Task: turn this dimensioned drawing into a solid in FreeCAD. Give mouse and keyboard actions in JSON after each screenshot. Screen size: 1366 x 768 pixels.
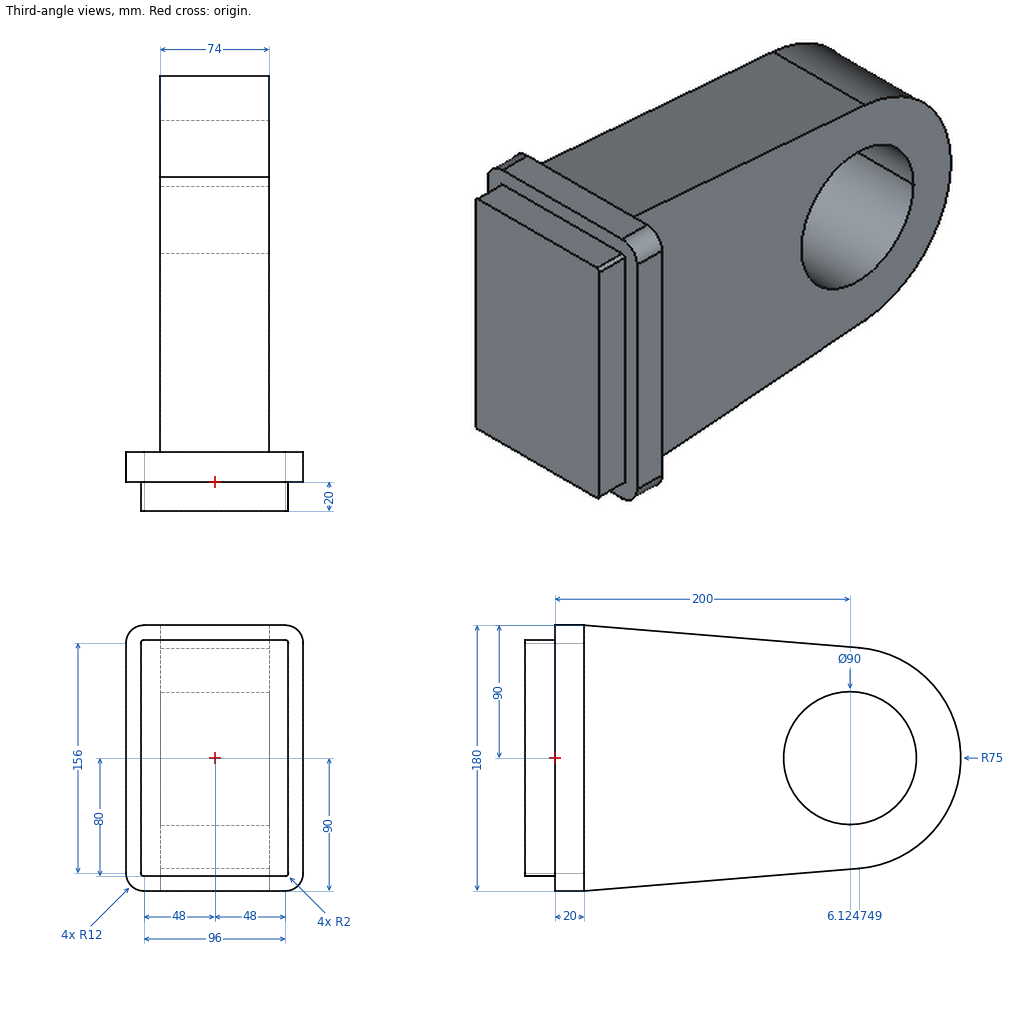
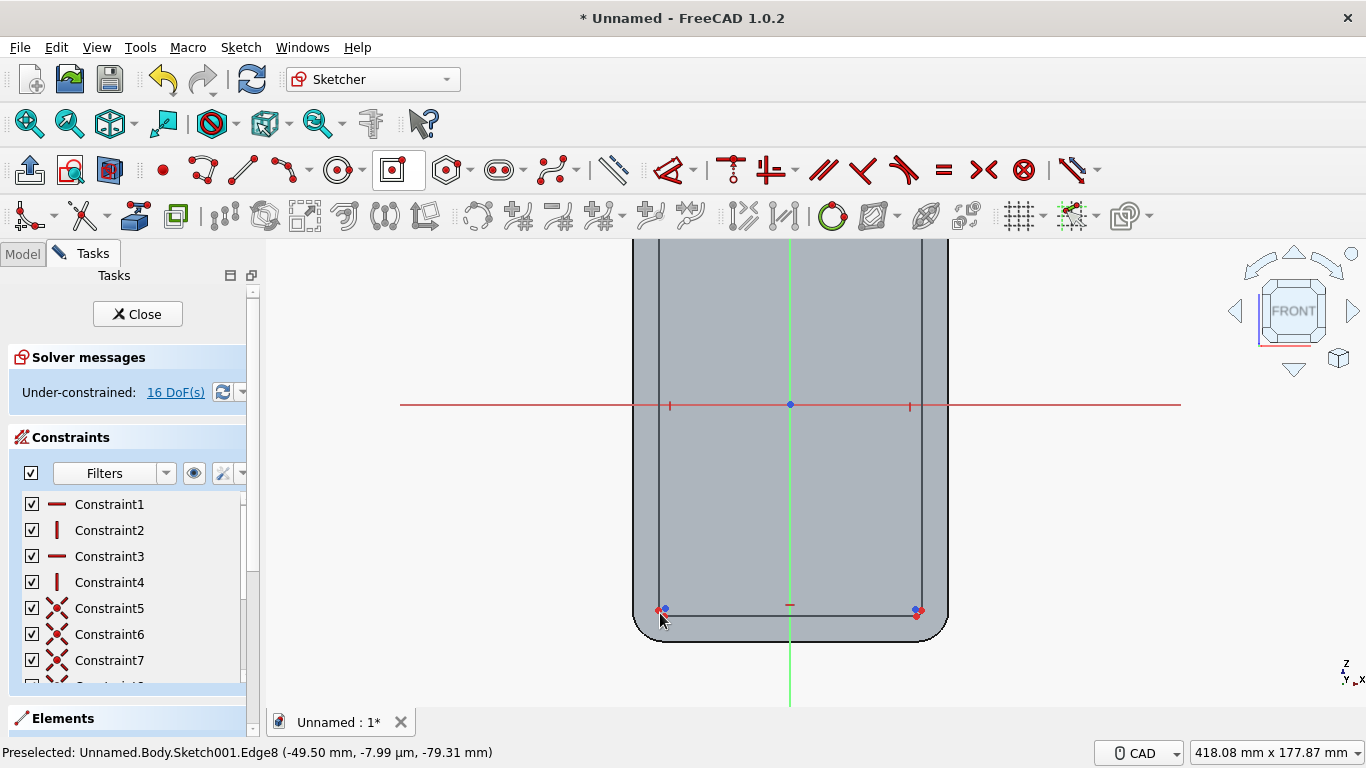
{"action": "left_click", "coordinate": [714, 615]}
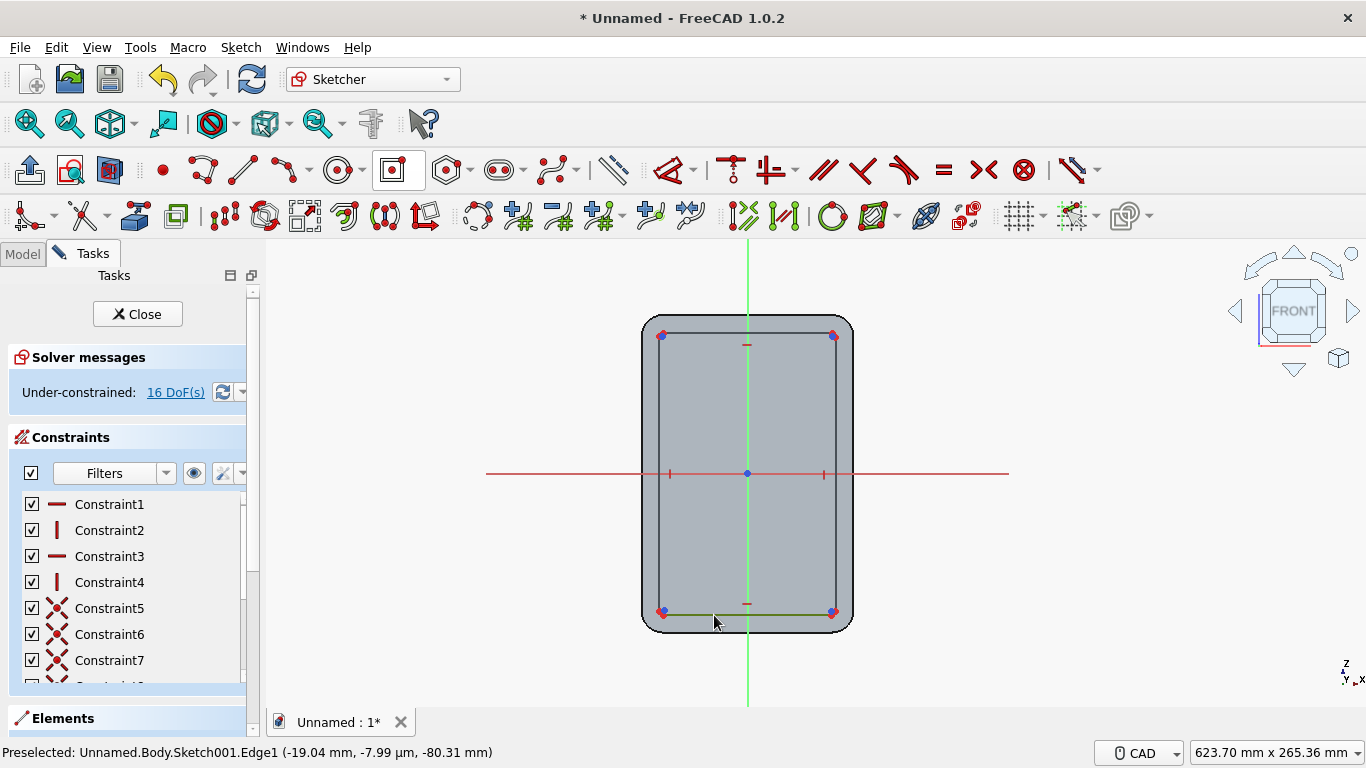
{"action": "scroll", "coordinate": [834, 614], "scroll_direction": "up", "scroll_amount": 9}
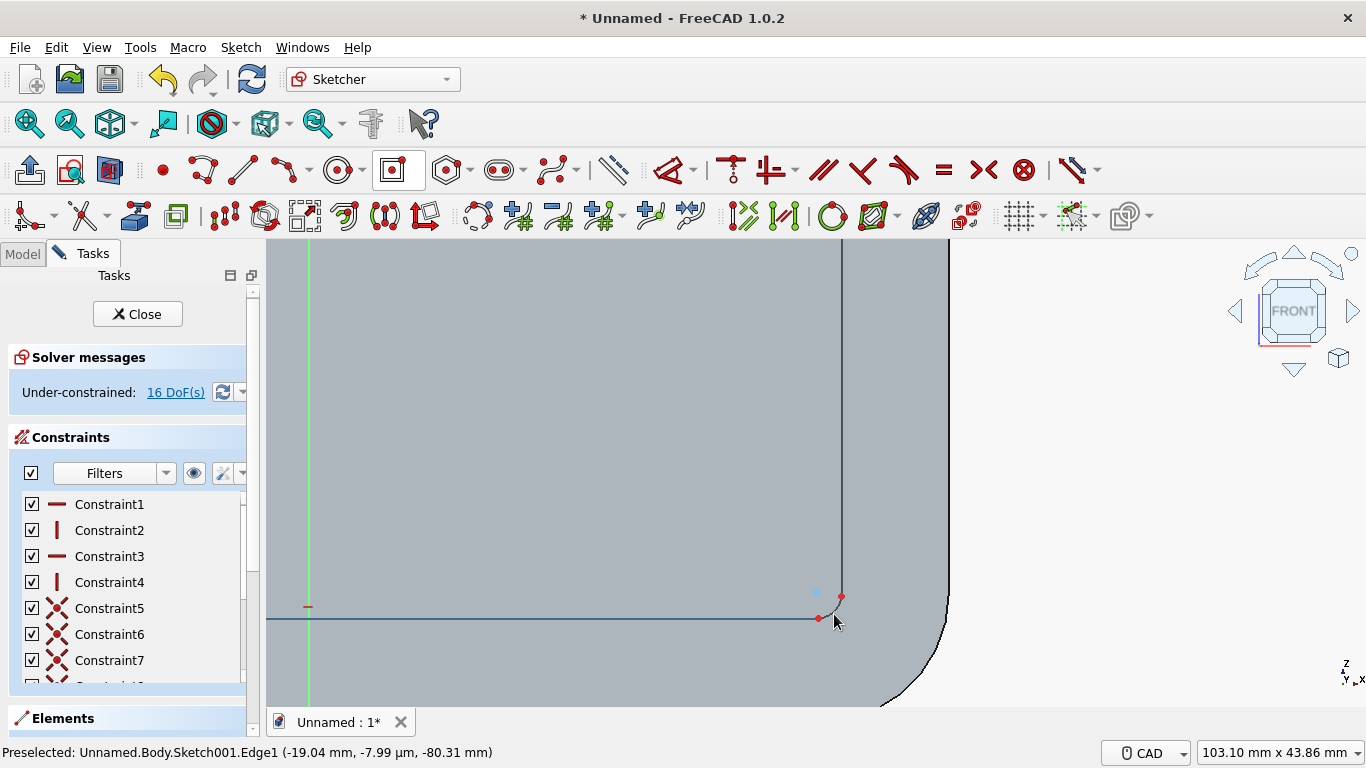
{"action": "left_click", "coordinate": [834, 611]}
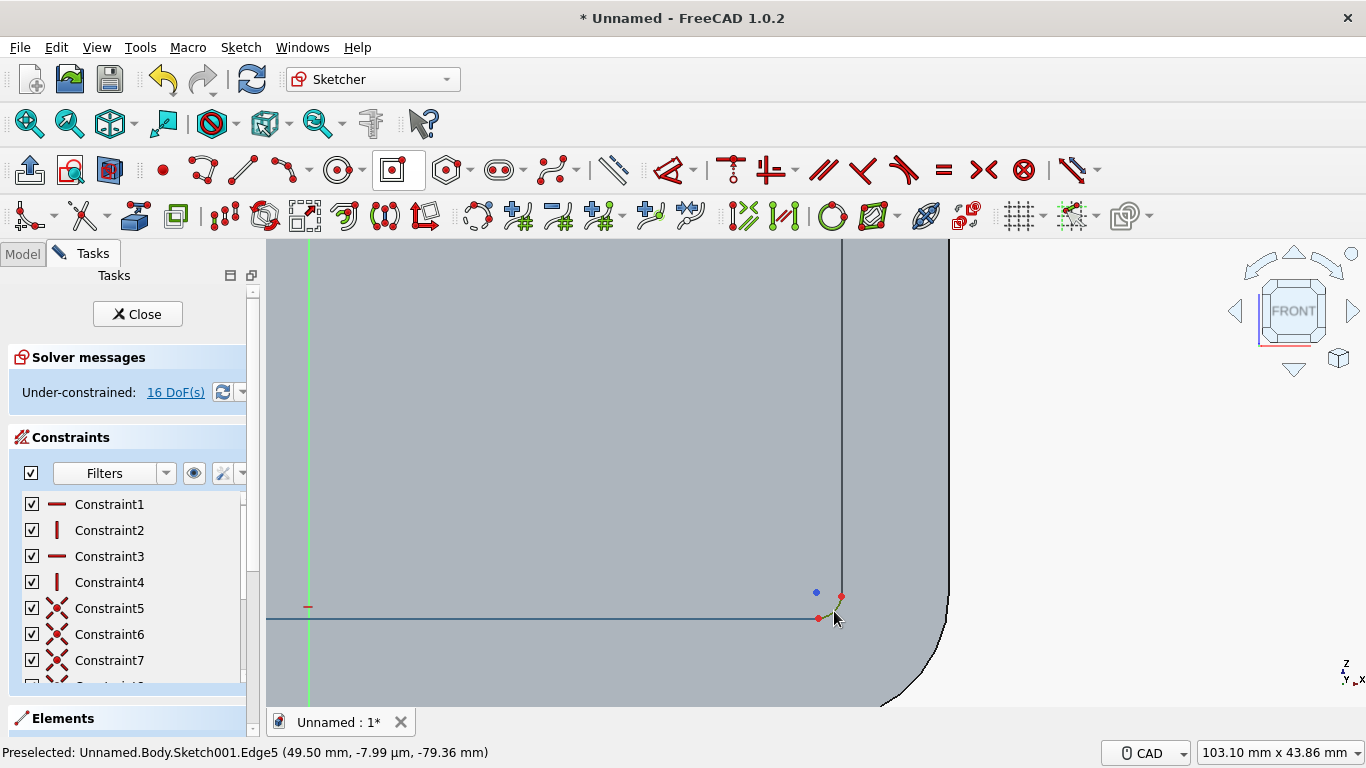
{"action": "key", "text": "t"}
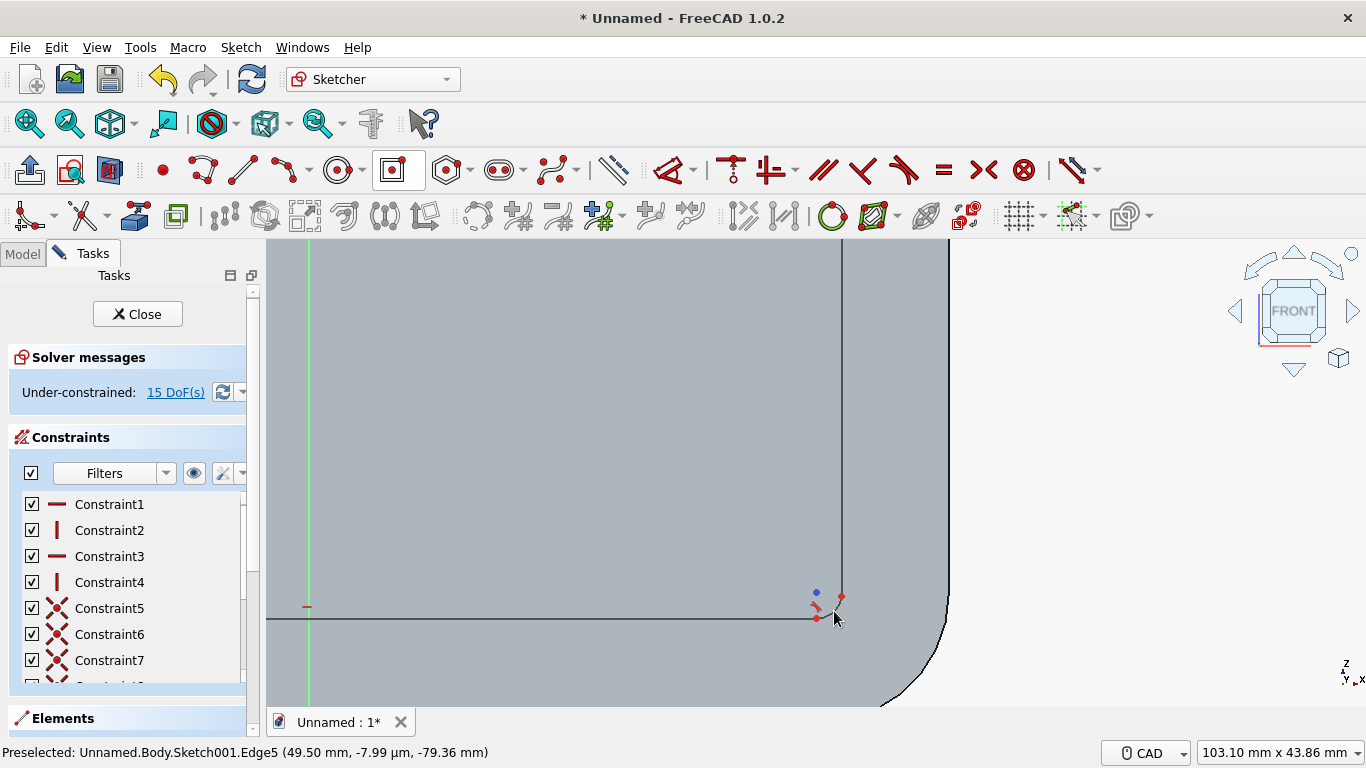
{"action": "scroll", "coordinate": [834, 614], "scroll_direction": "down", "scroll_amount": 9}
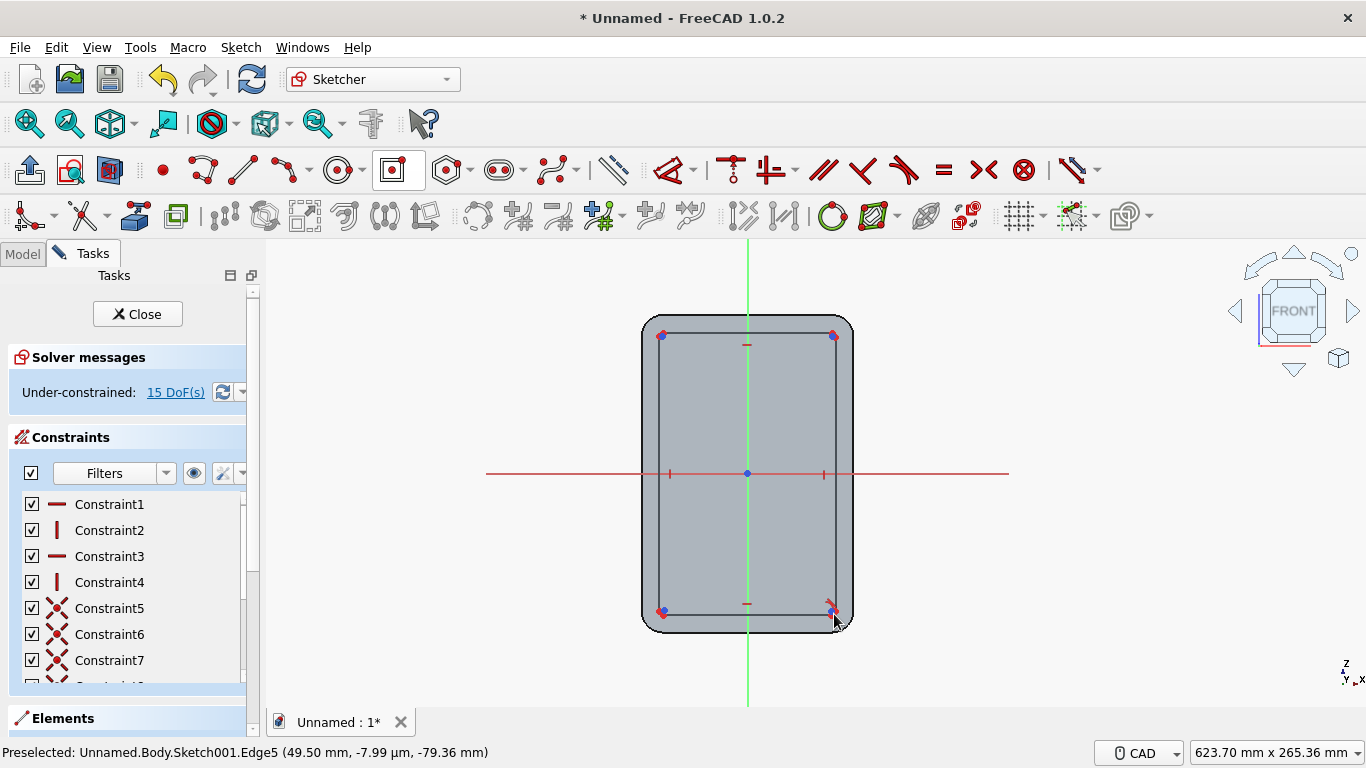
{"action": "left_click", "coordinate": [781, 615]}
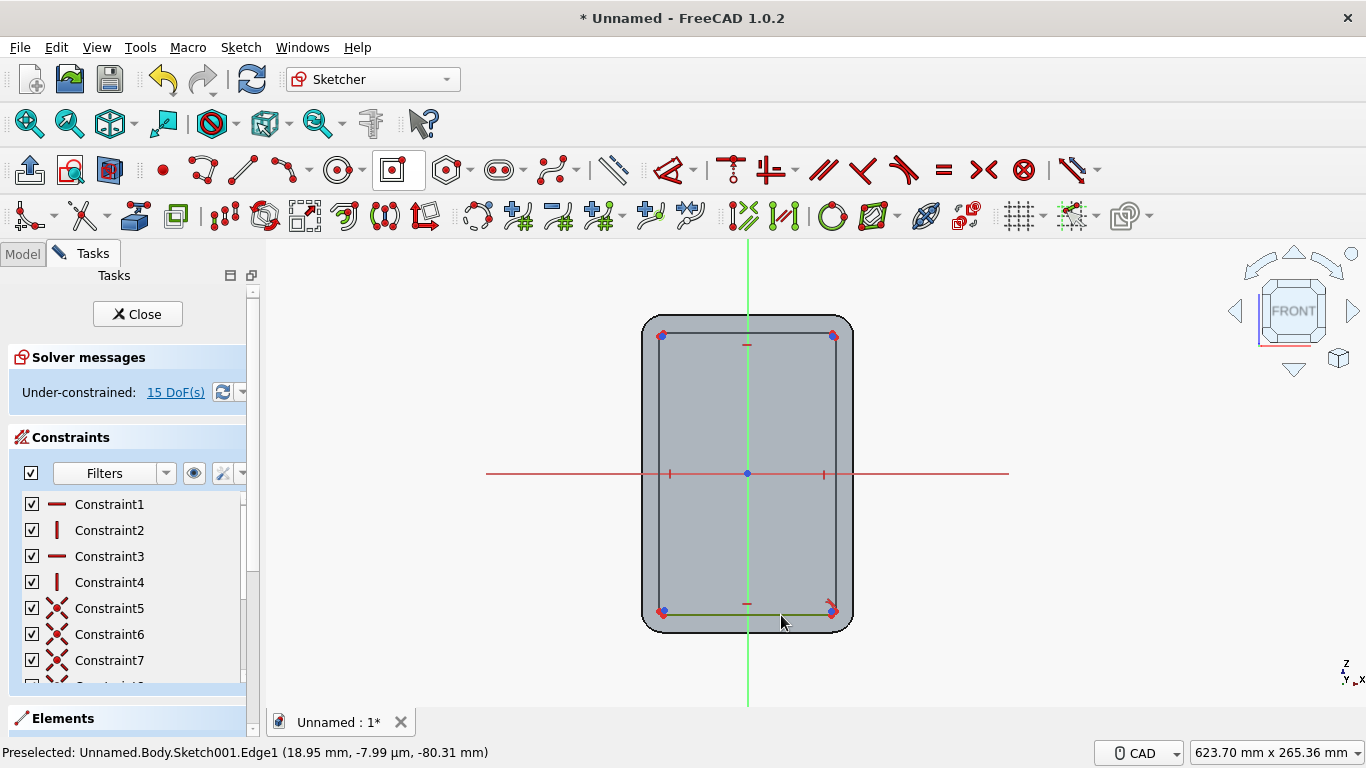
{"action": "scroll", "coordinate": [661, 614], "scroll_direction": "up", "scroll_amount": 8}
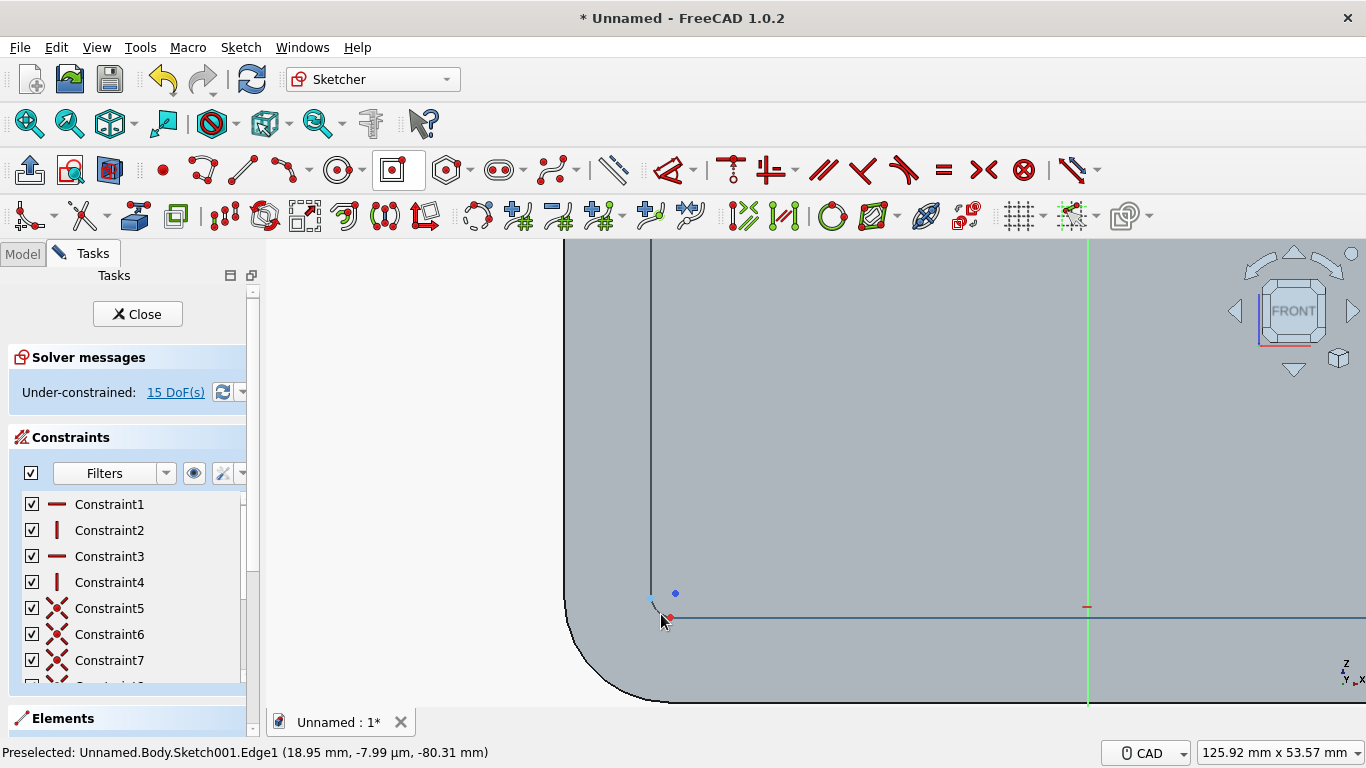
{"action": "left_click", "coordinate": [658, 611]}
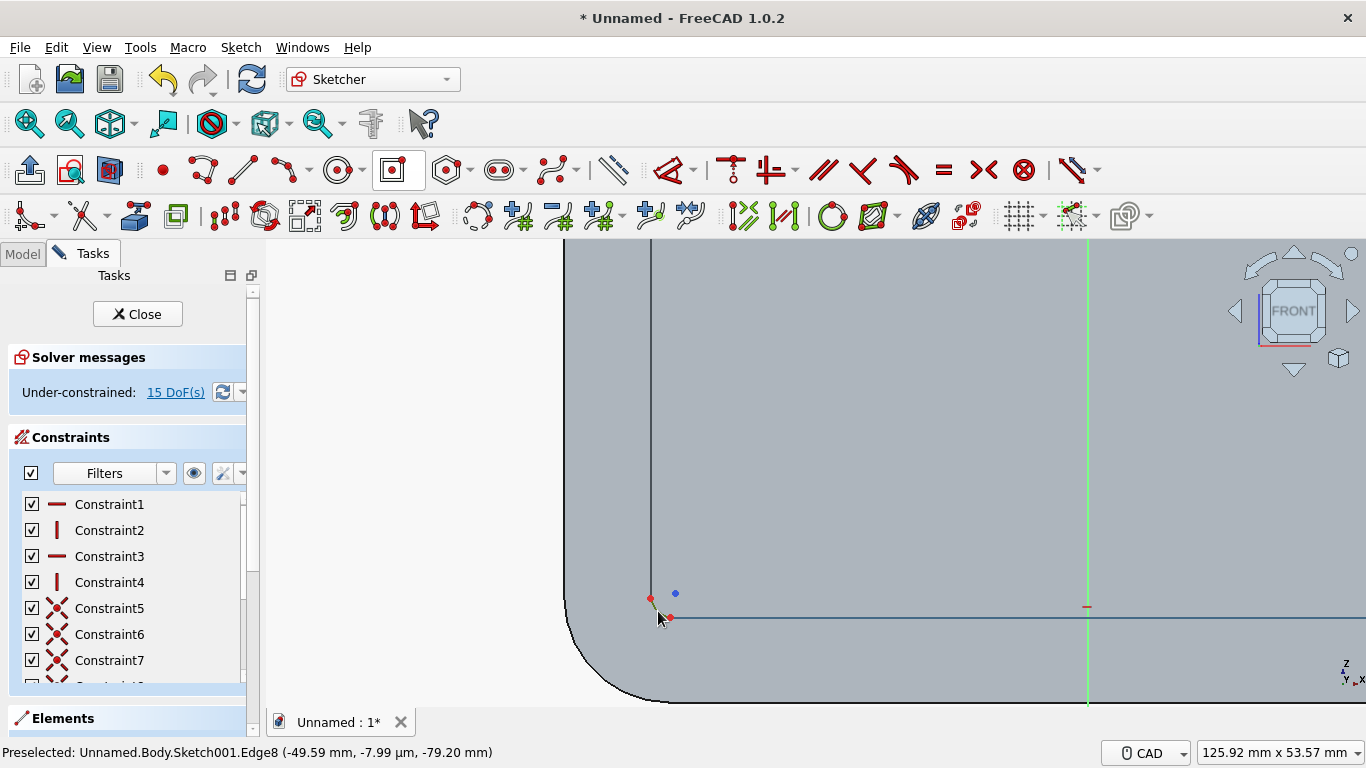
{"action": "left_click", "coordinate": [904, 170]}